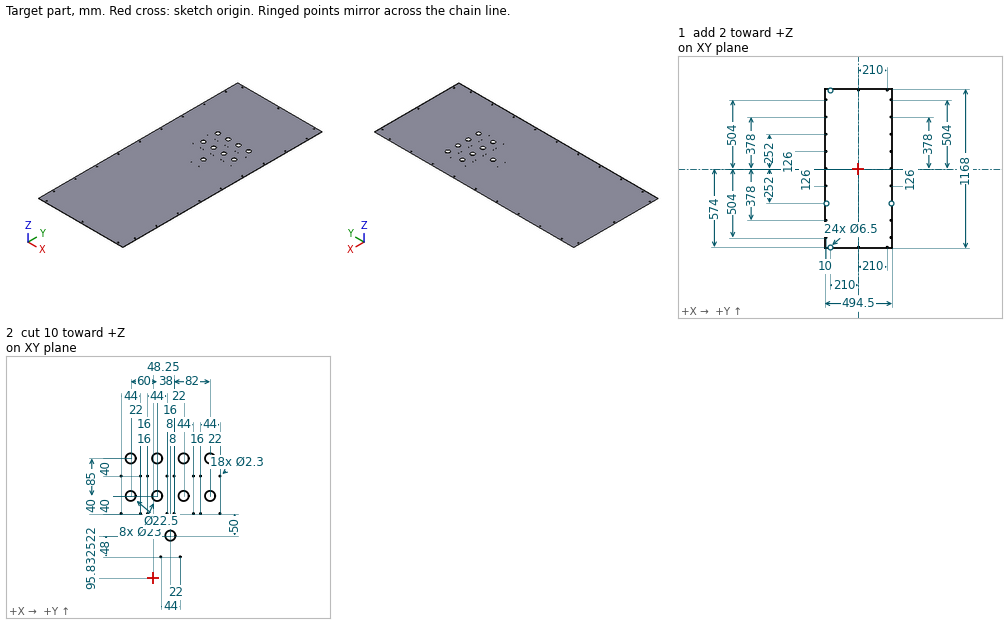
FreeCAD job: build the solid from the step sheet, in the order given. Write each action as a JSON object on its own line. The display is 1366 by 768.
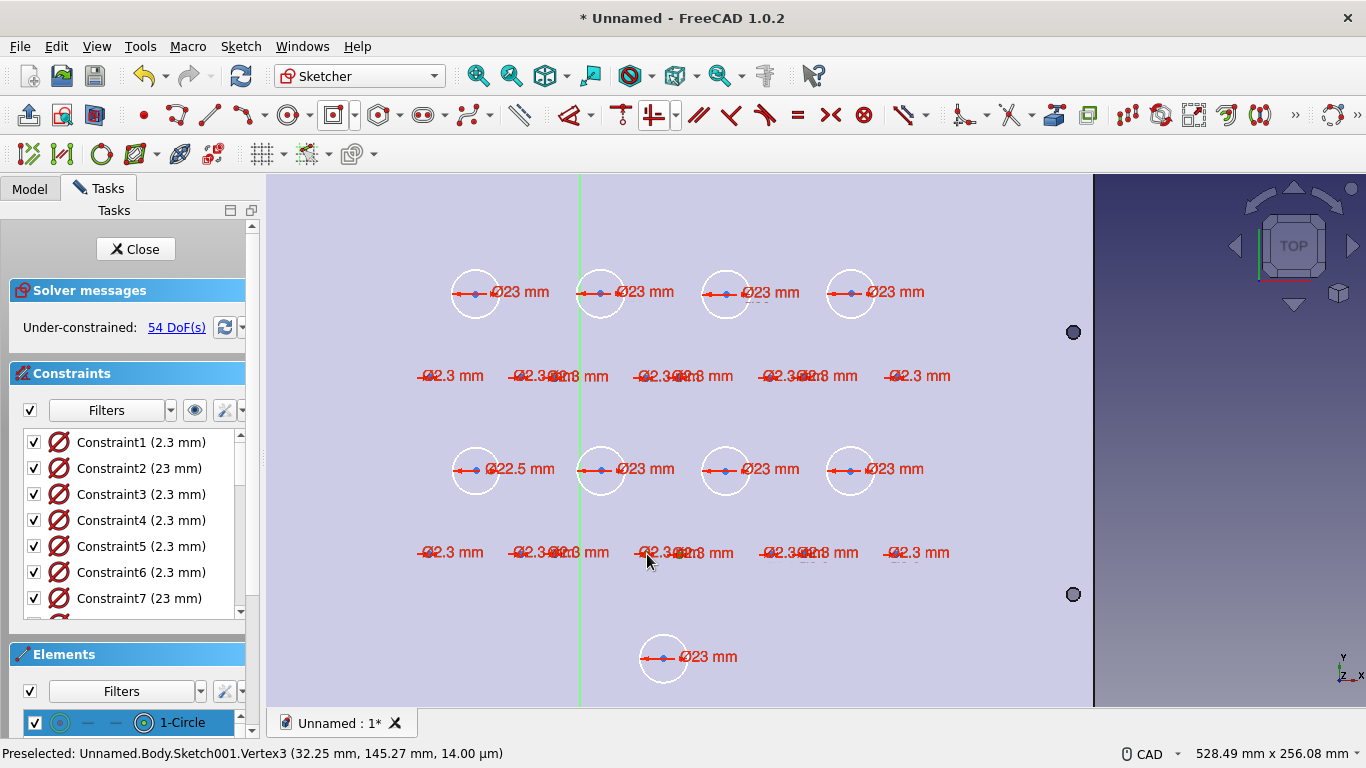
{"action": "left_click", "coordinate": [676, 116]}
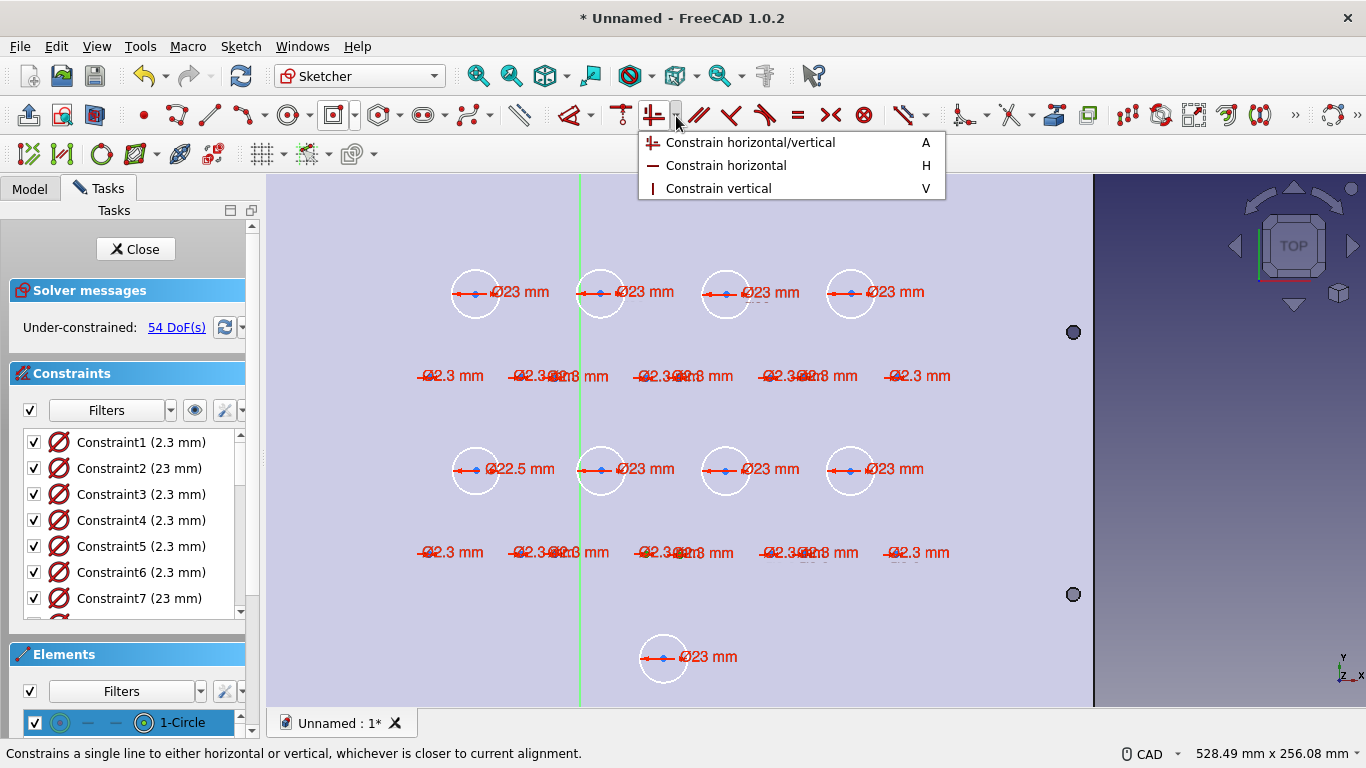
{"action": "left_click", "coordinate": [792, 166]}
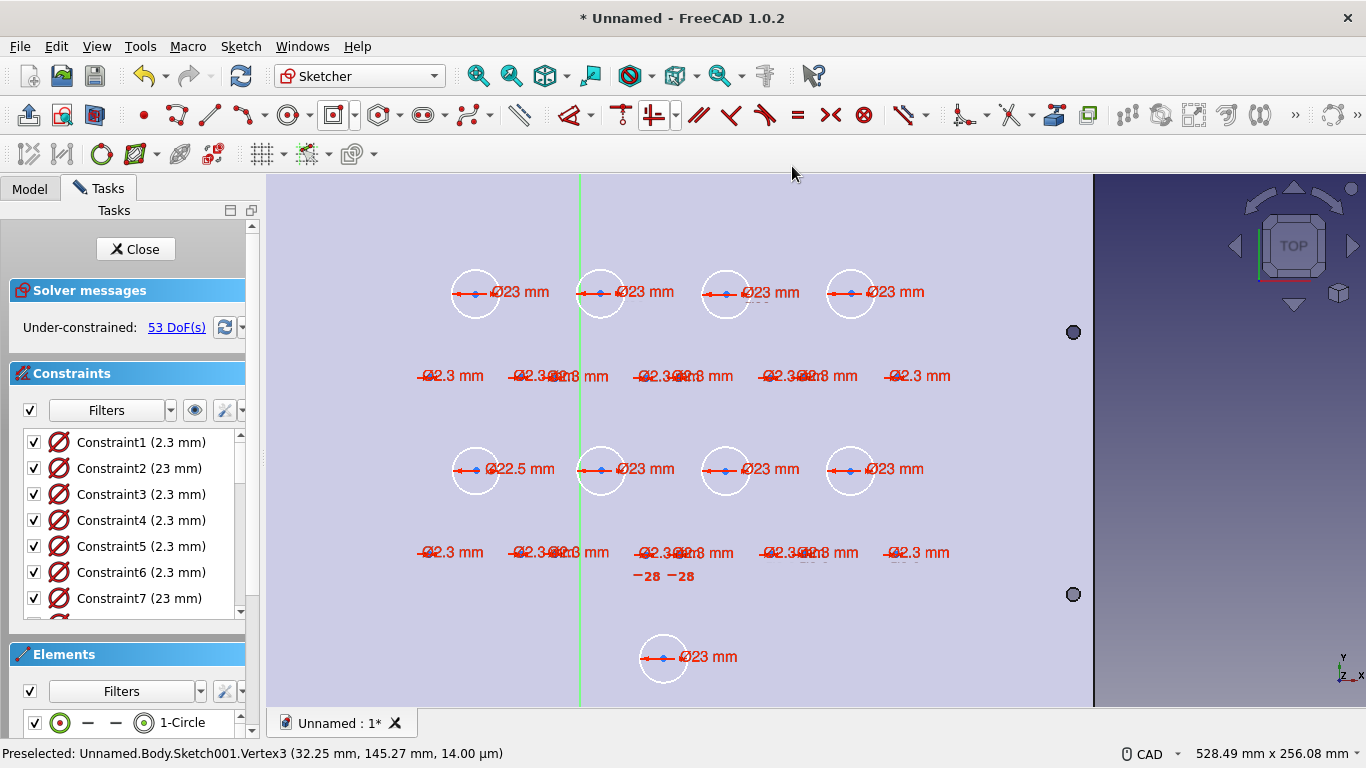
{"action": "left_click", "coordinate": [647, 555]}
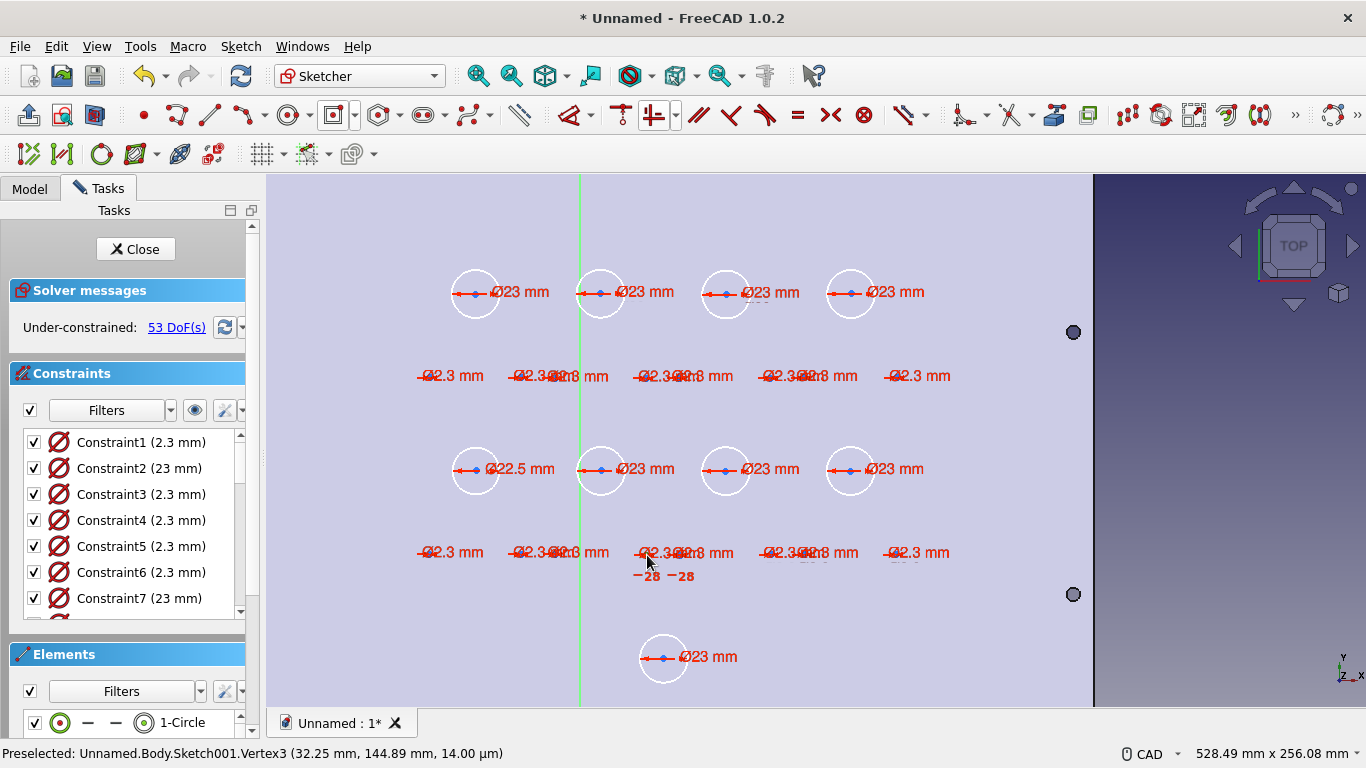
{"action": "left_click", "coordinate": [556, 554]}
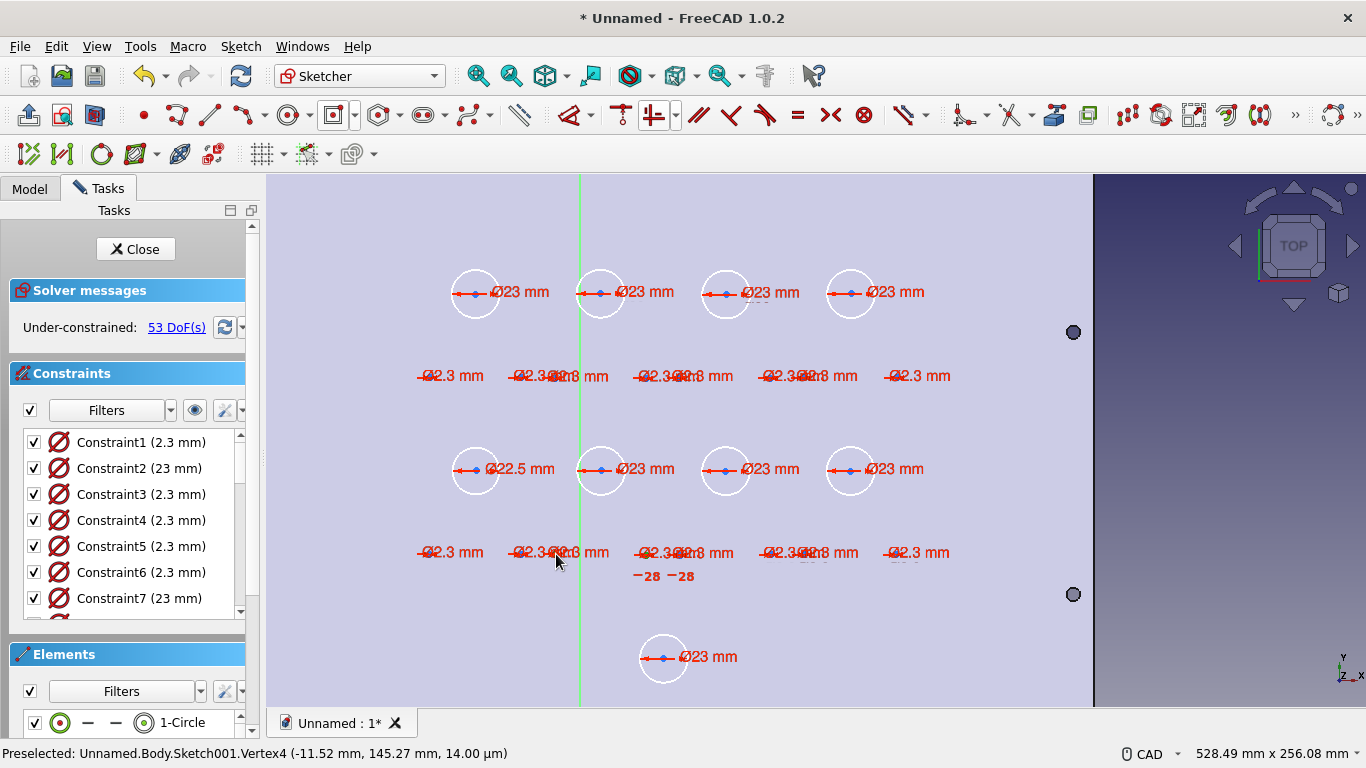
{"action": "key", "text": "h"}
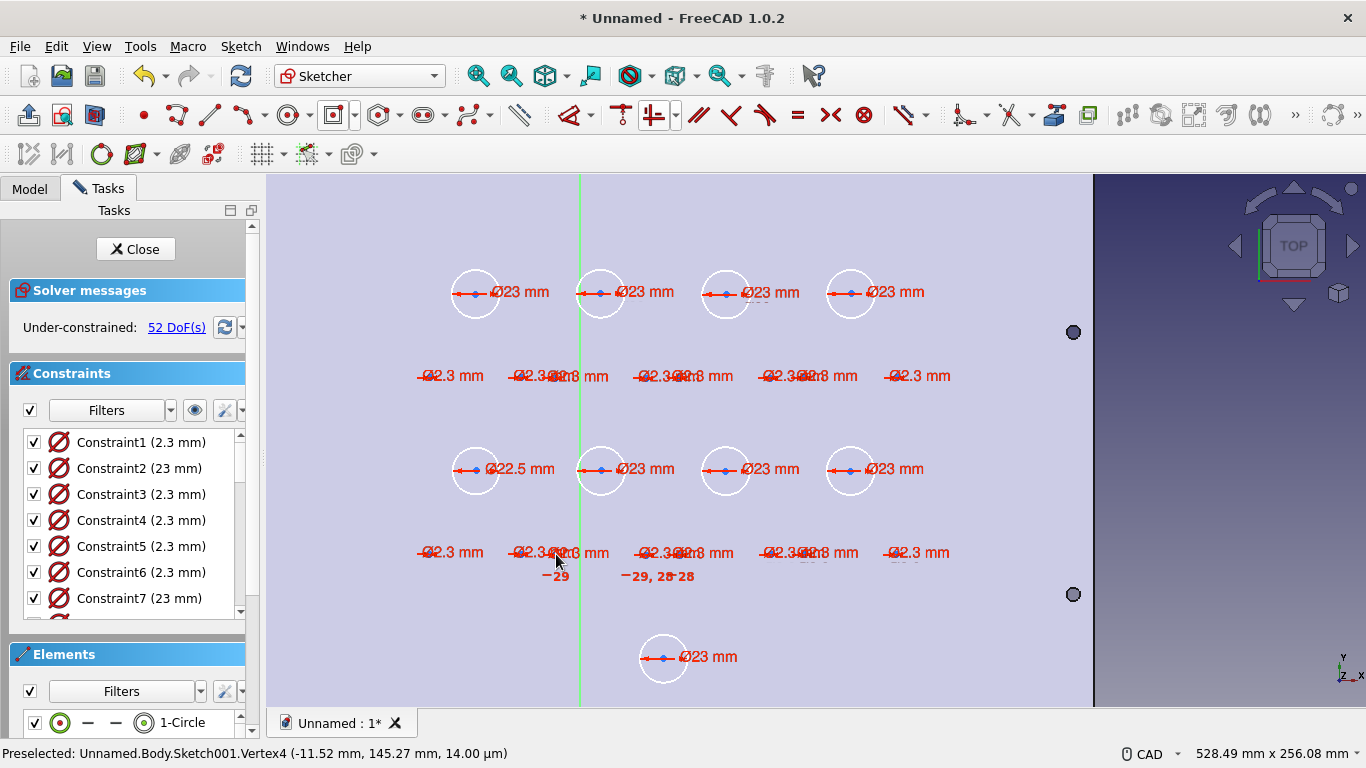
{"action": "left_click", "coordinate": [556, 555]}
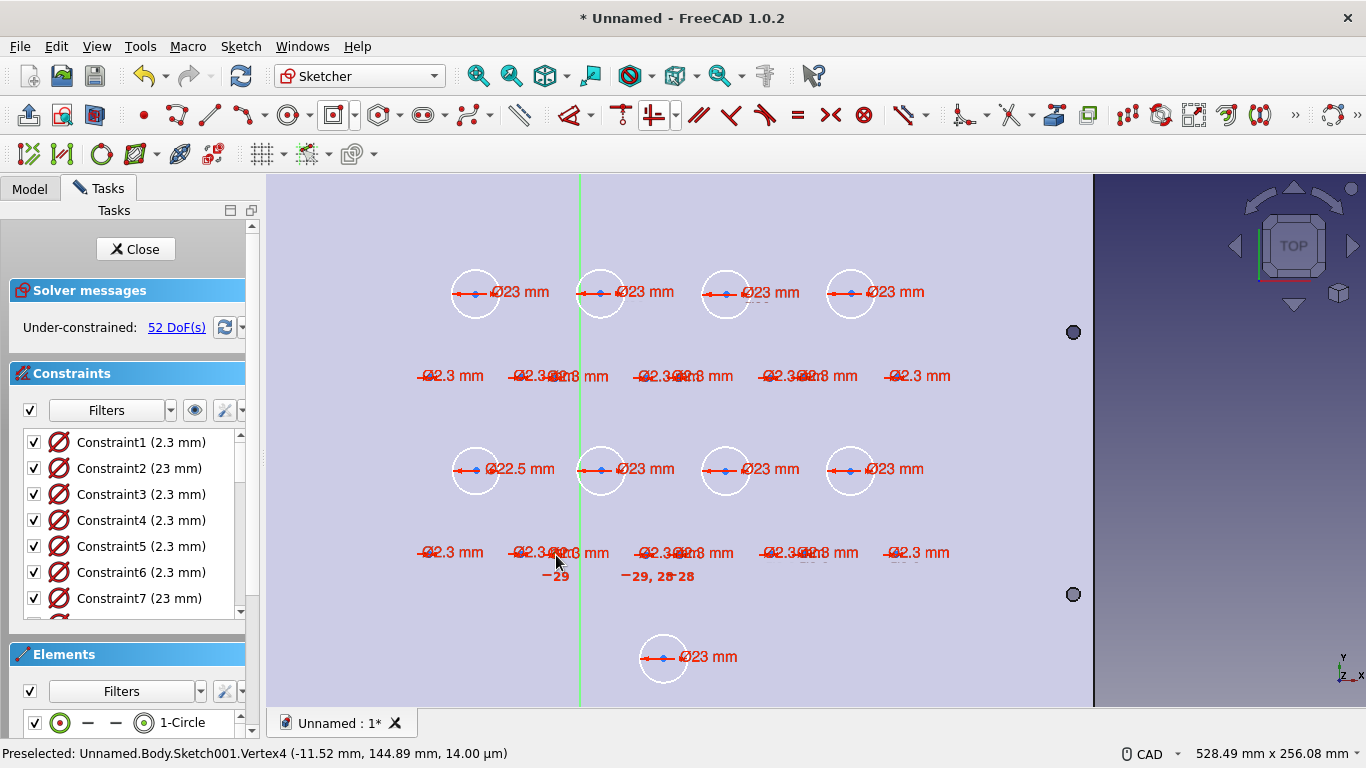
{"action": "left_click", "coordinate": [521, 554]}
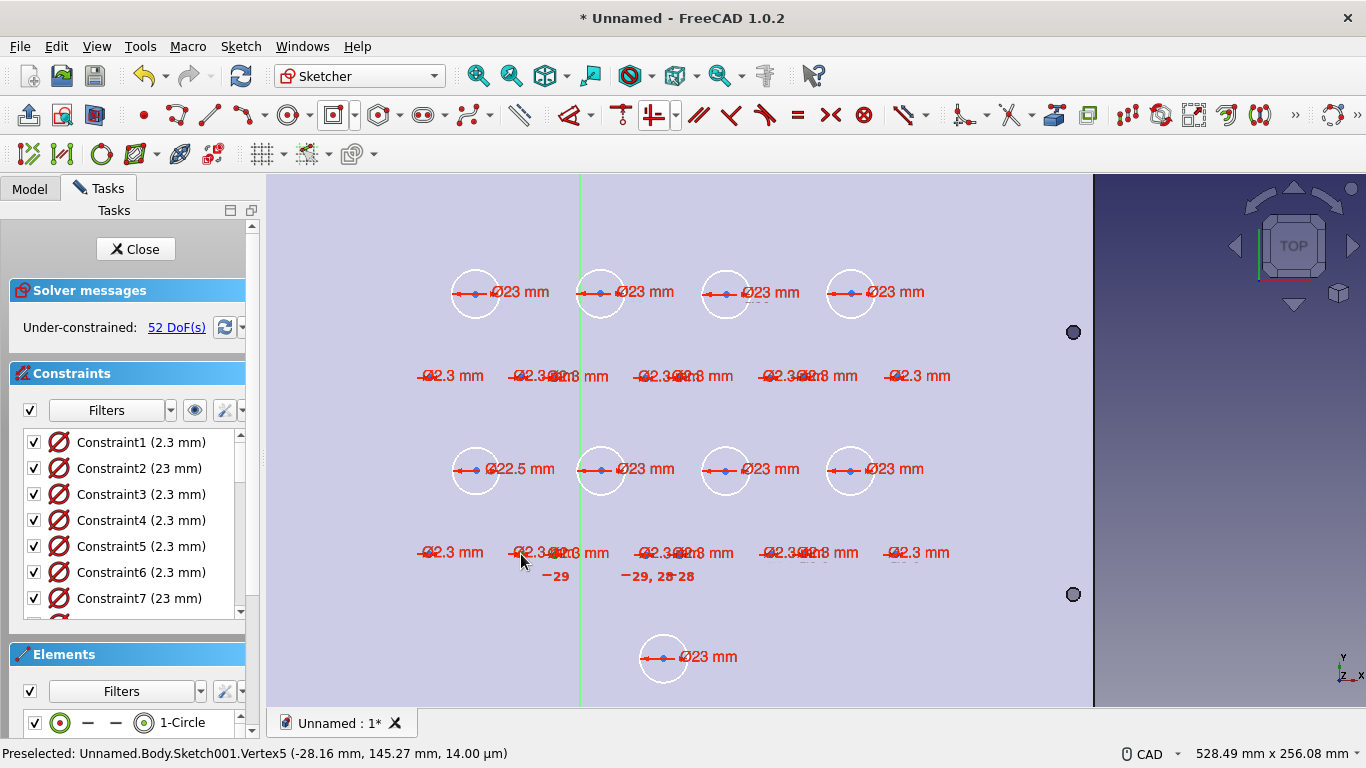
{"action": "left_click", "coordinate": [676, 116]}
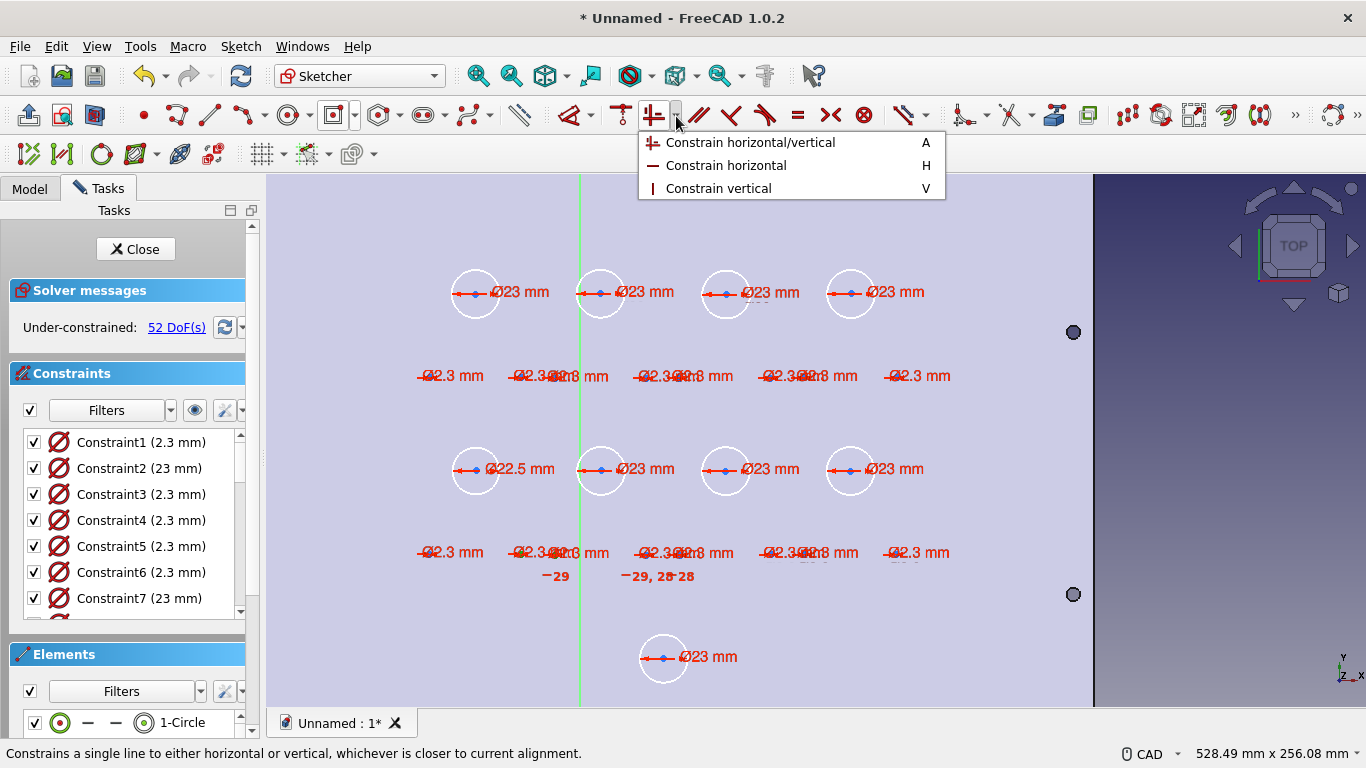
{"action": "left_click", "coordinate": [792, 166]}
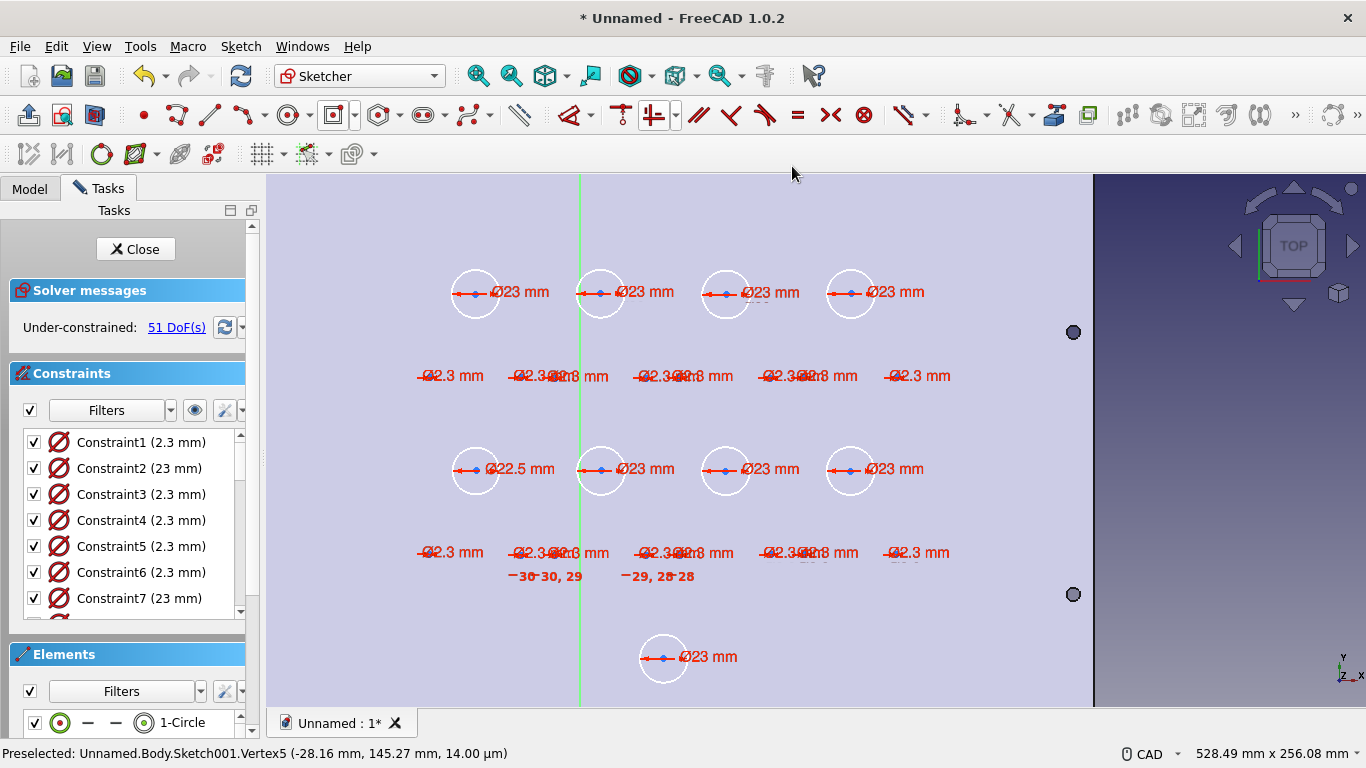
{"action": "left_click", "coordinate": [521, 555]}